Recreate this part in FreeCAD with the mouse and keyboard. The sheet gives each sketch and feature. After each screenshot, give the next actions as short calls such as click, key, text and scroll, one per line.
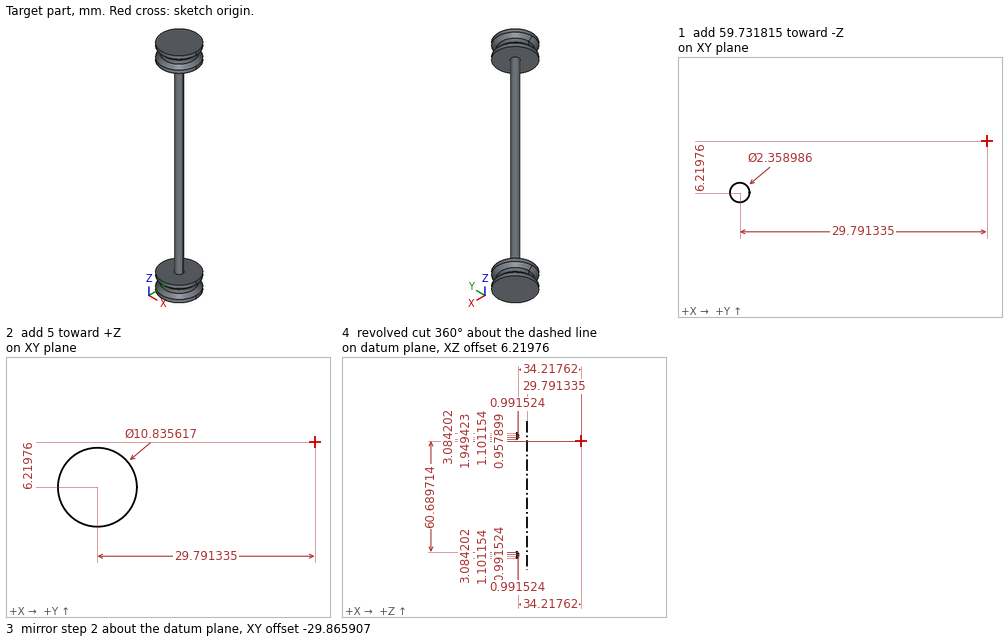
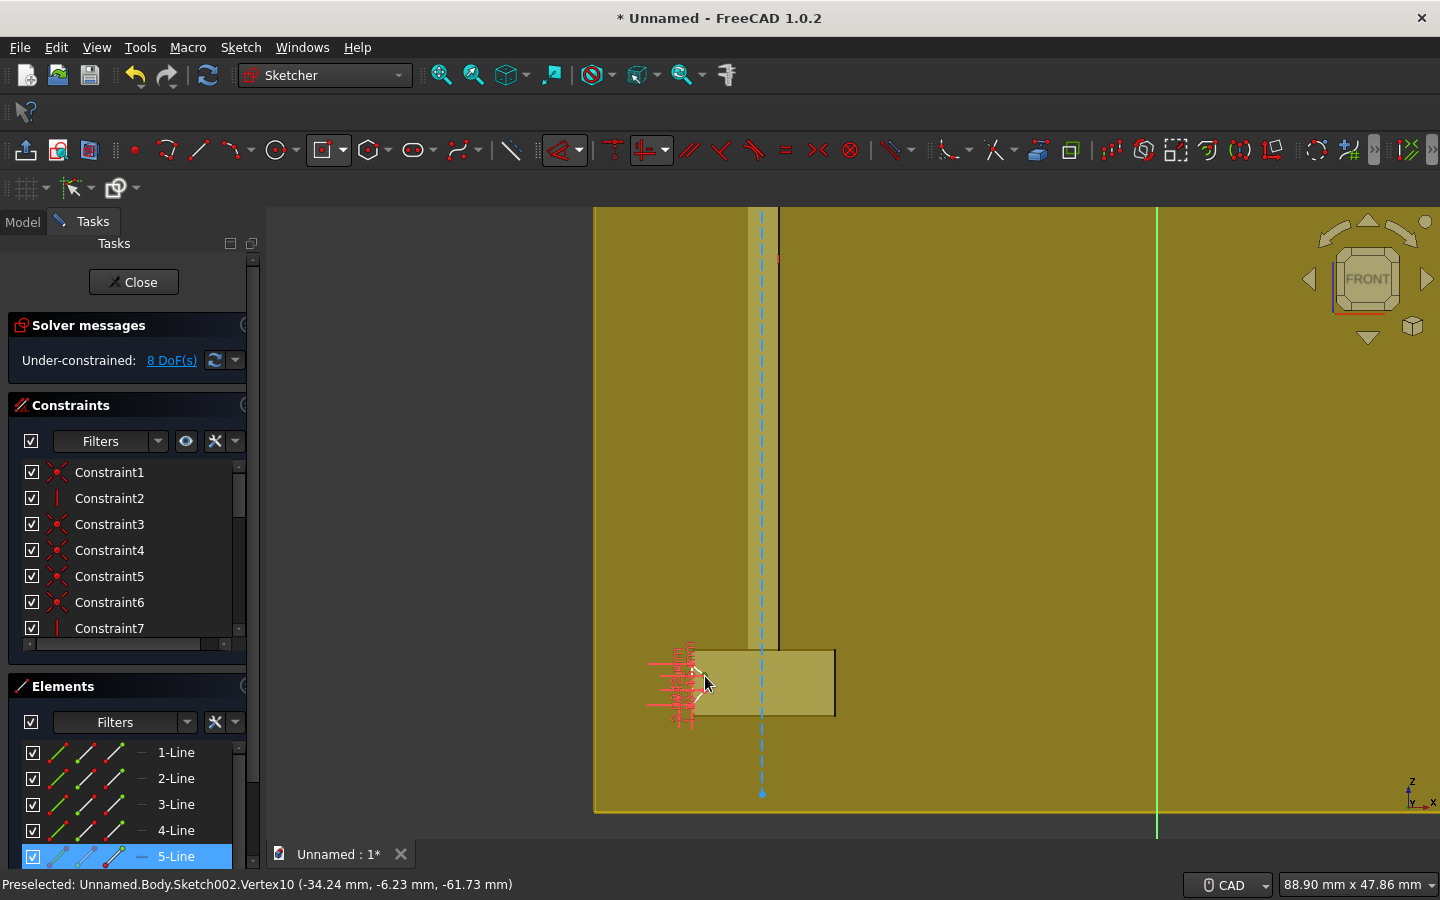
key(l)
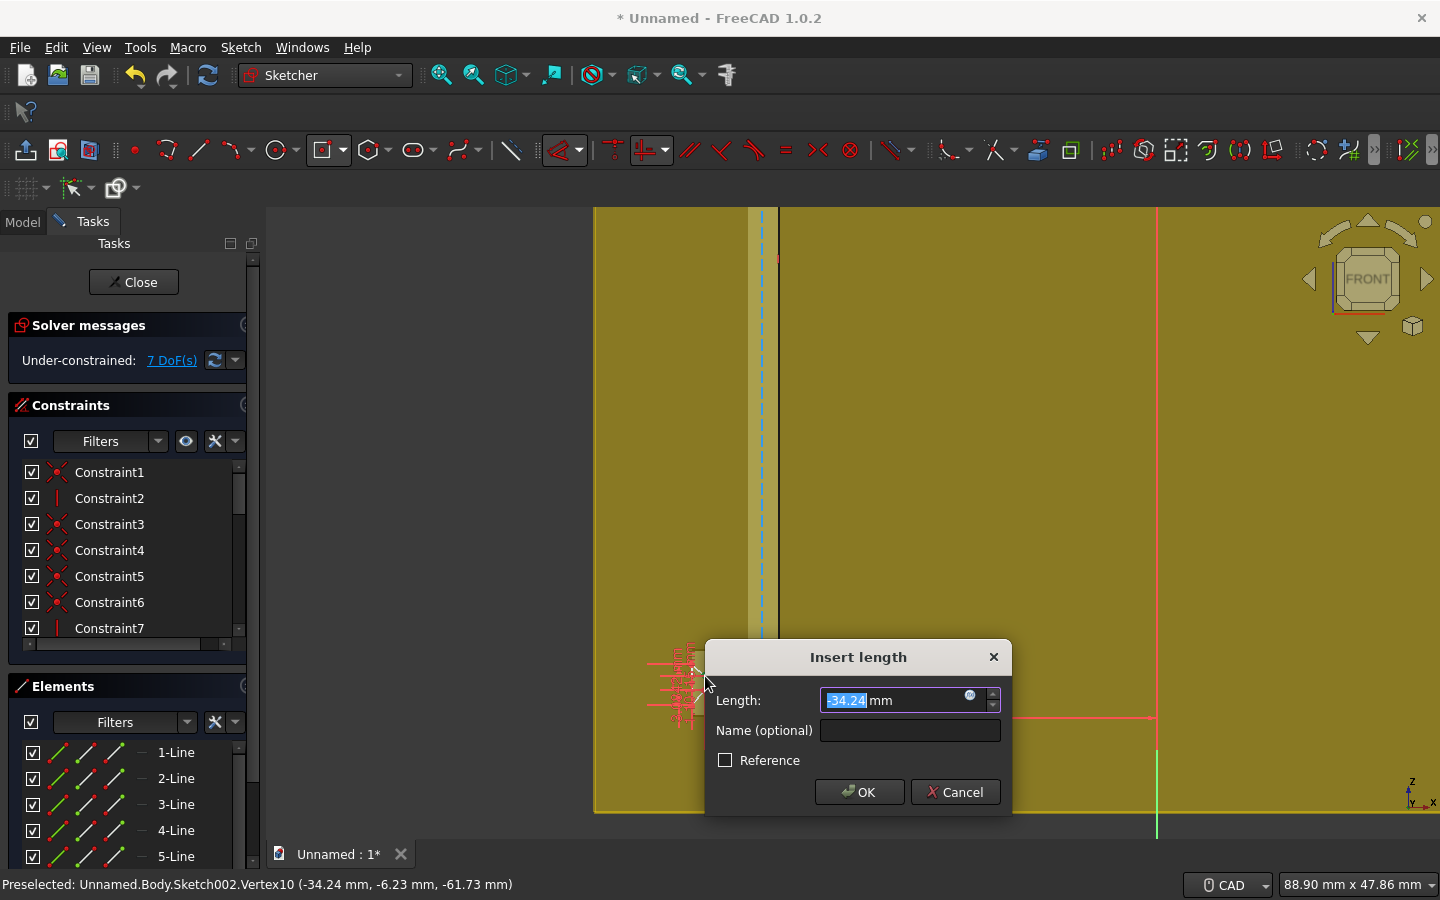
text(-34.21762)
key(Return)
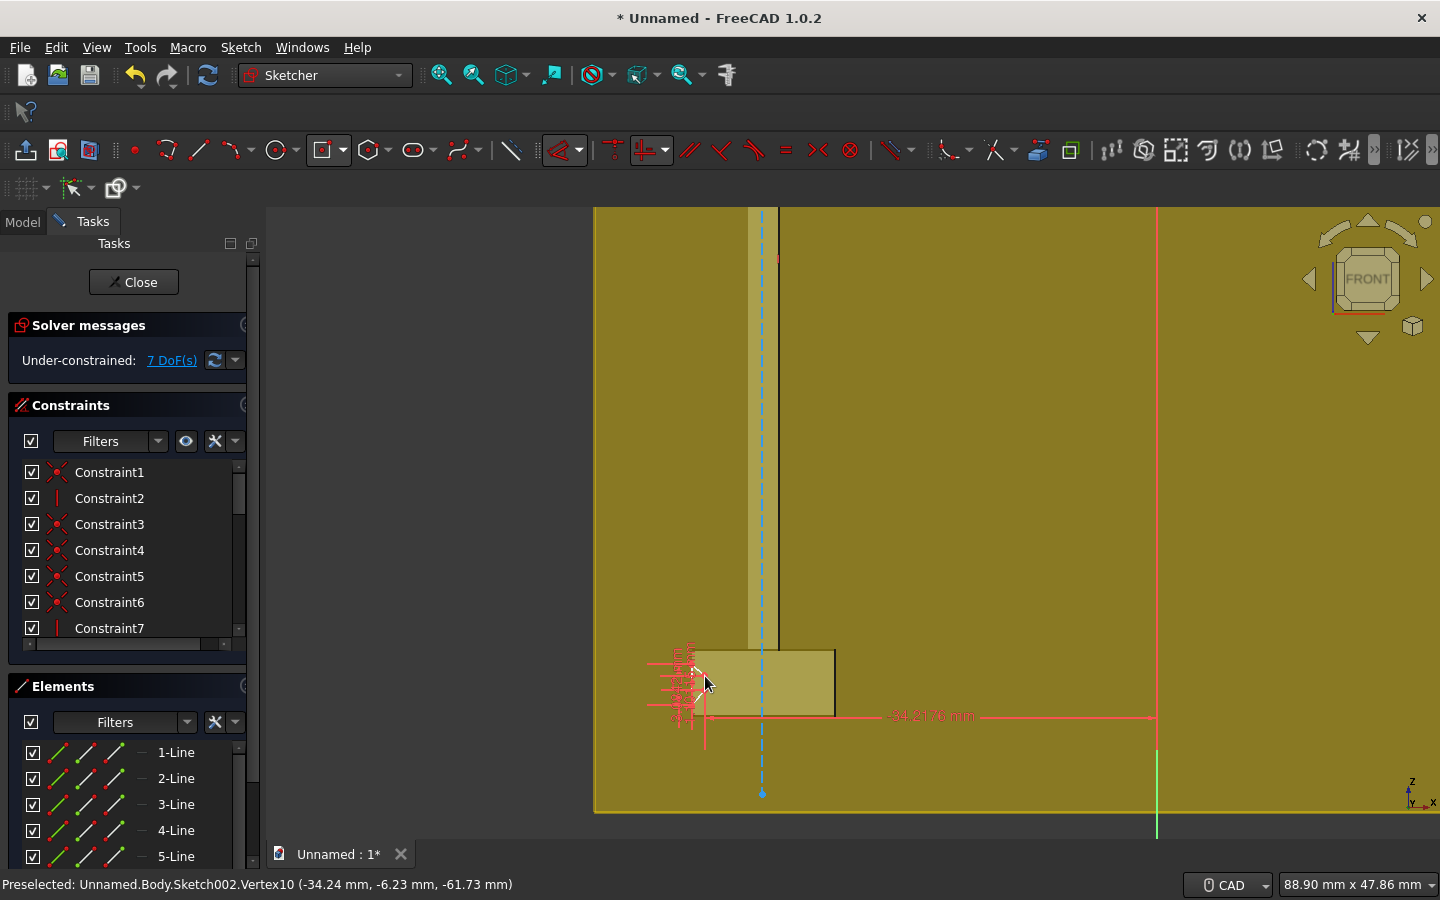
scroll(703, 679, down, 5)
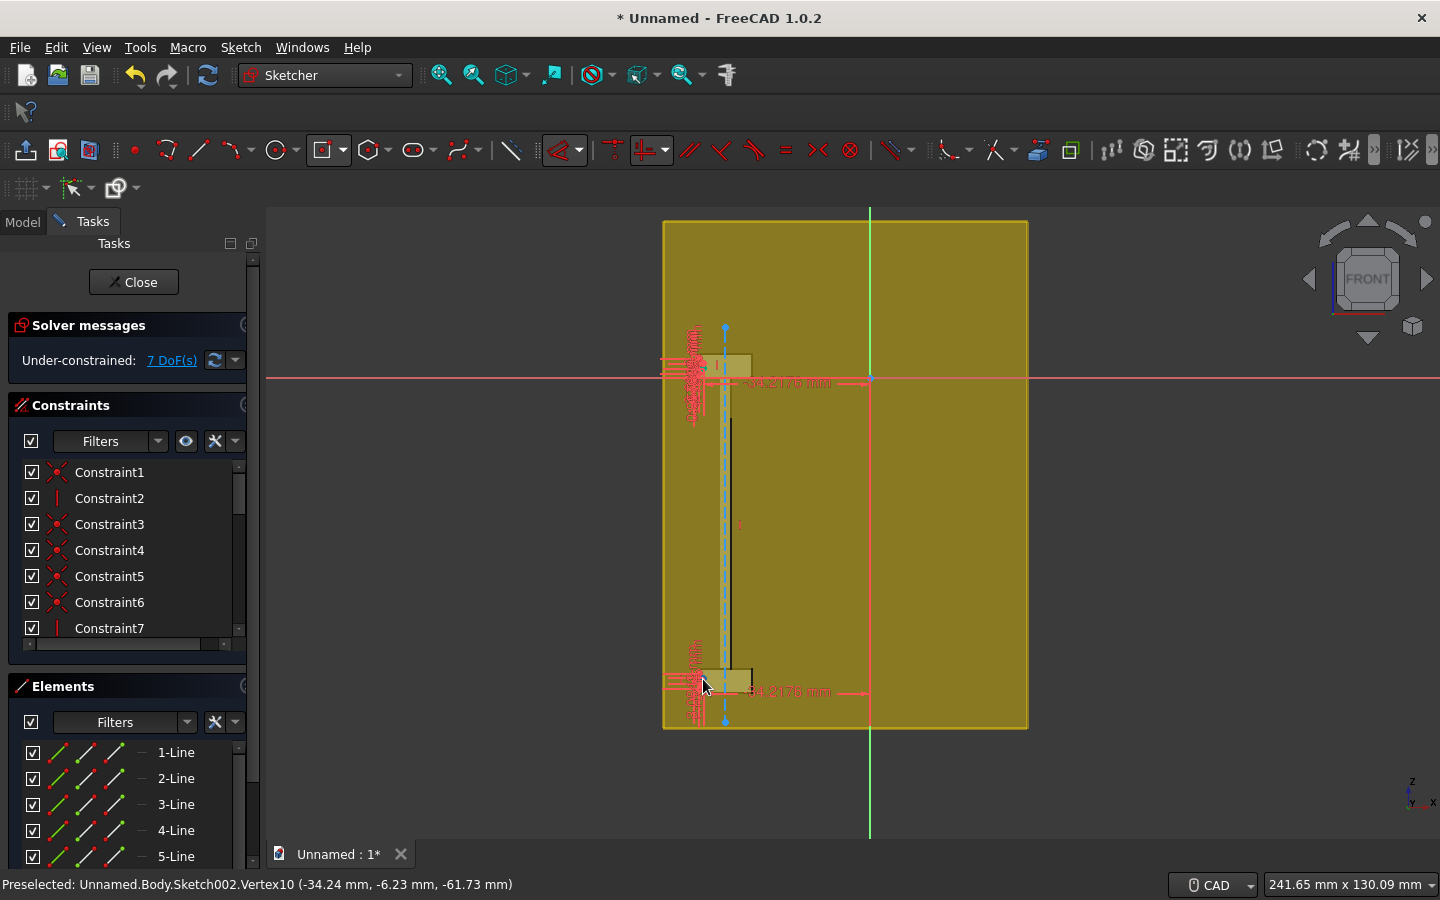
scroll(702, 371, up, 11)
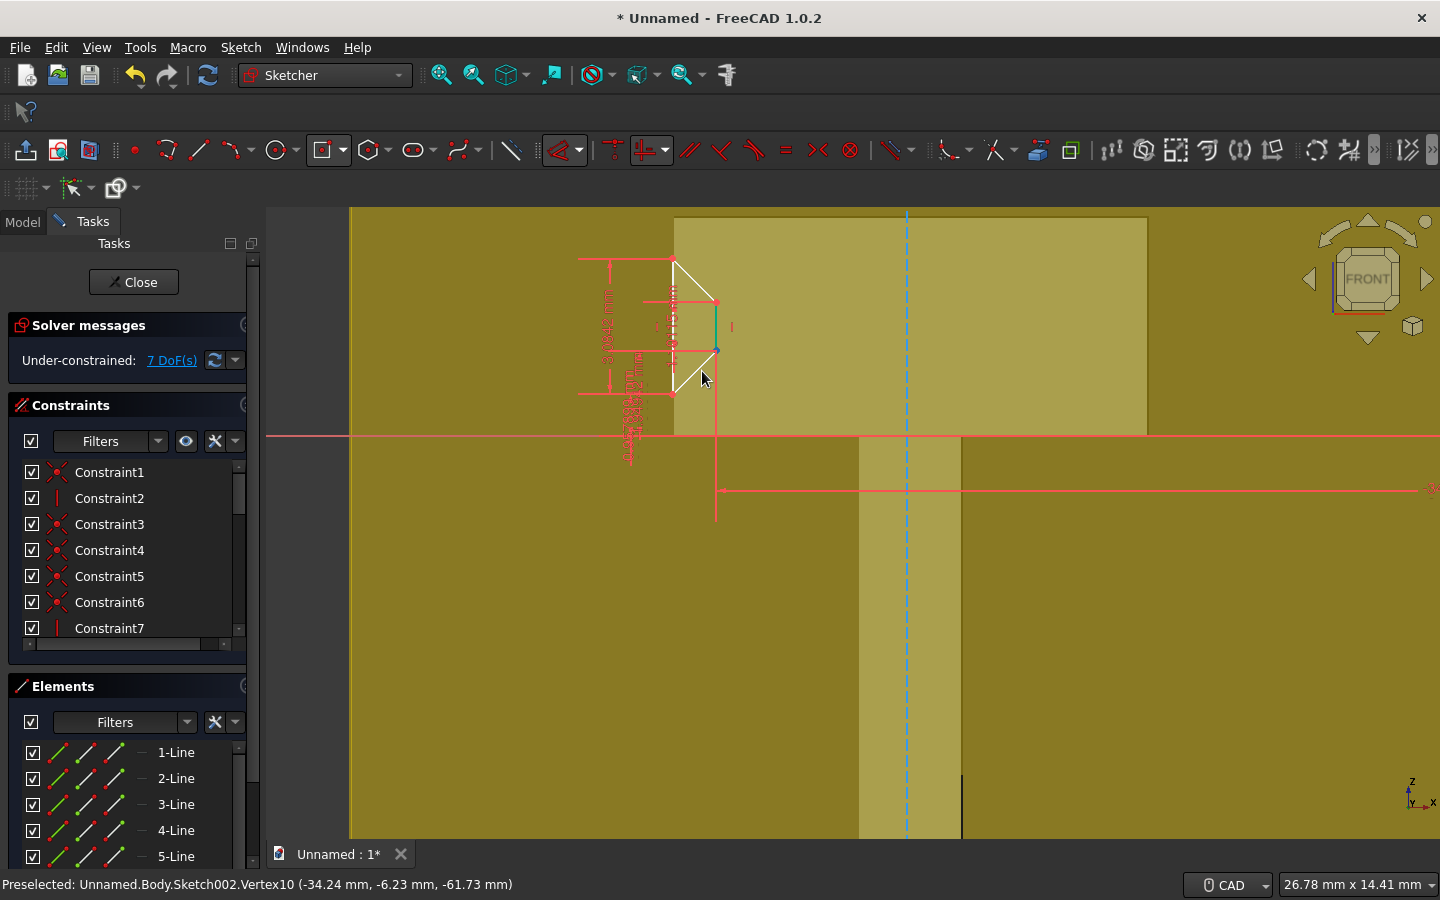
click(699, 368)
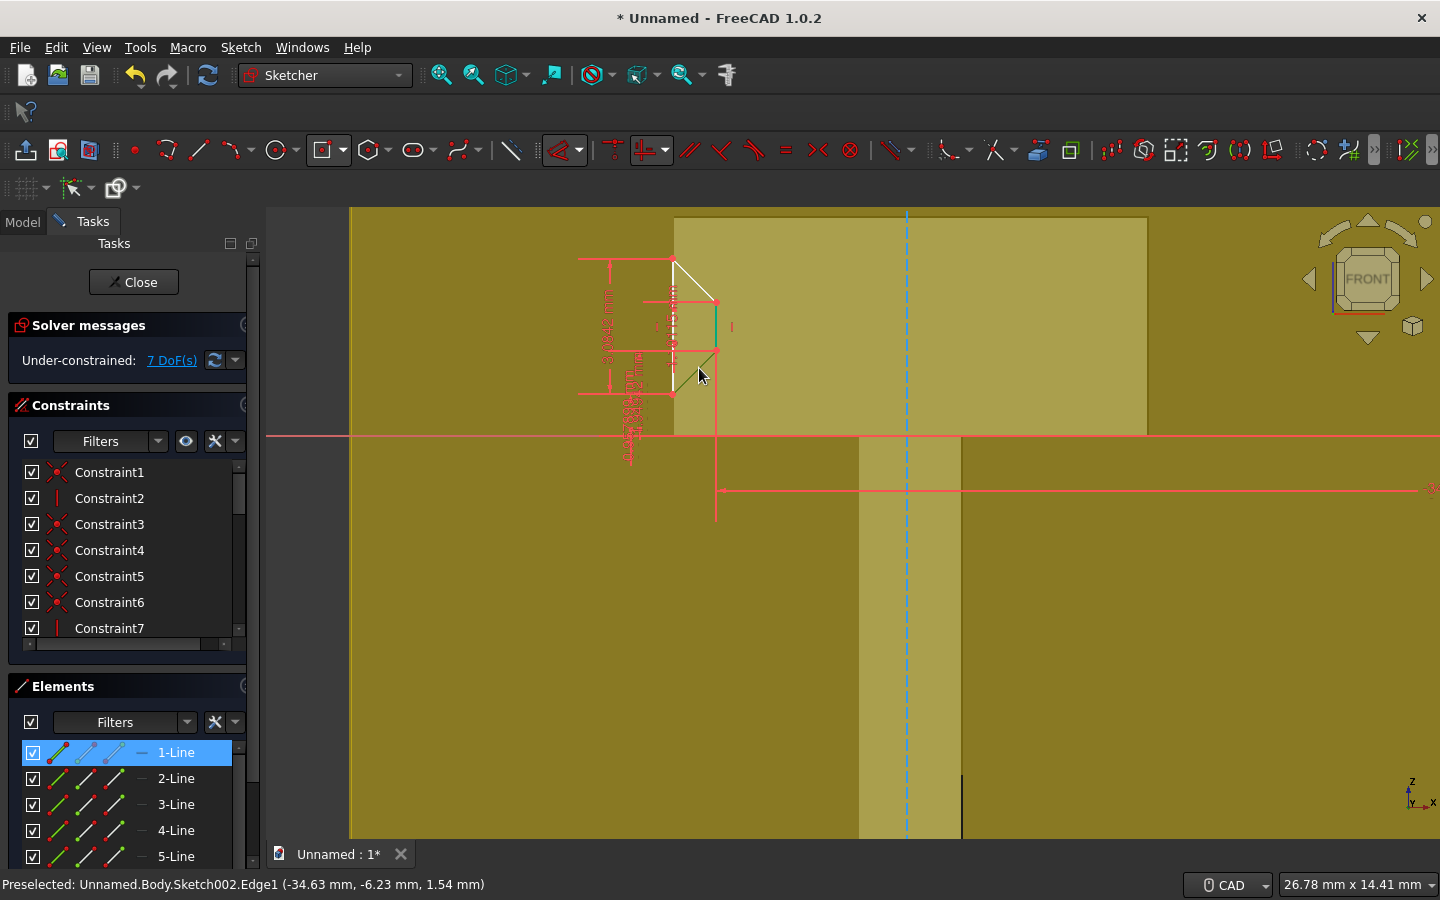
key(l)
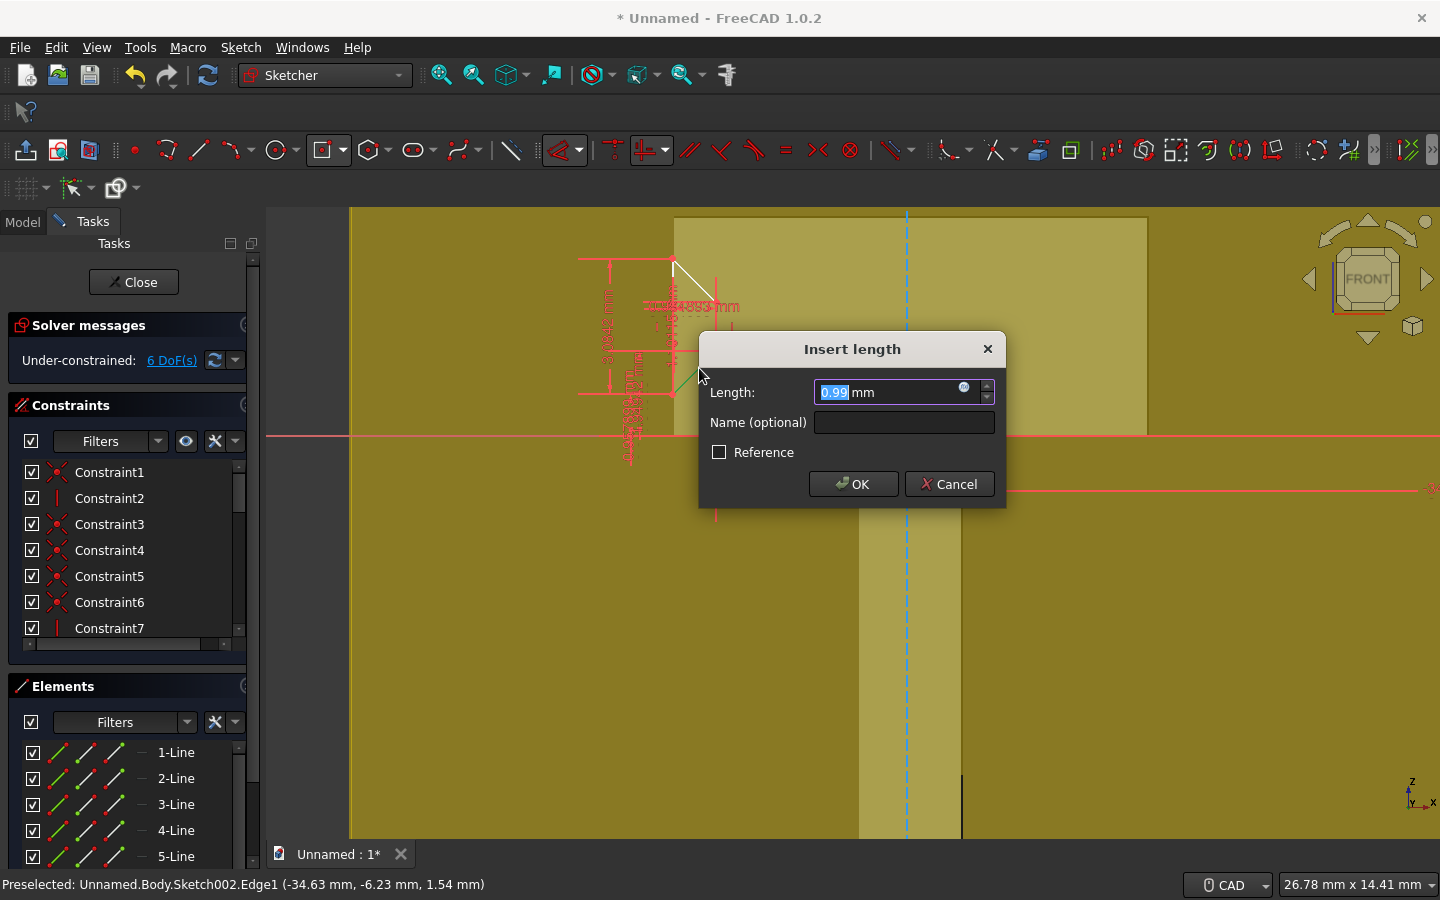
text(0.991524)
key(Return)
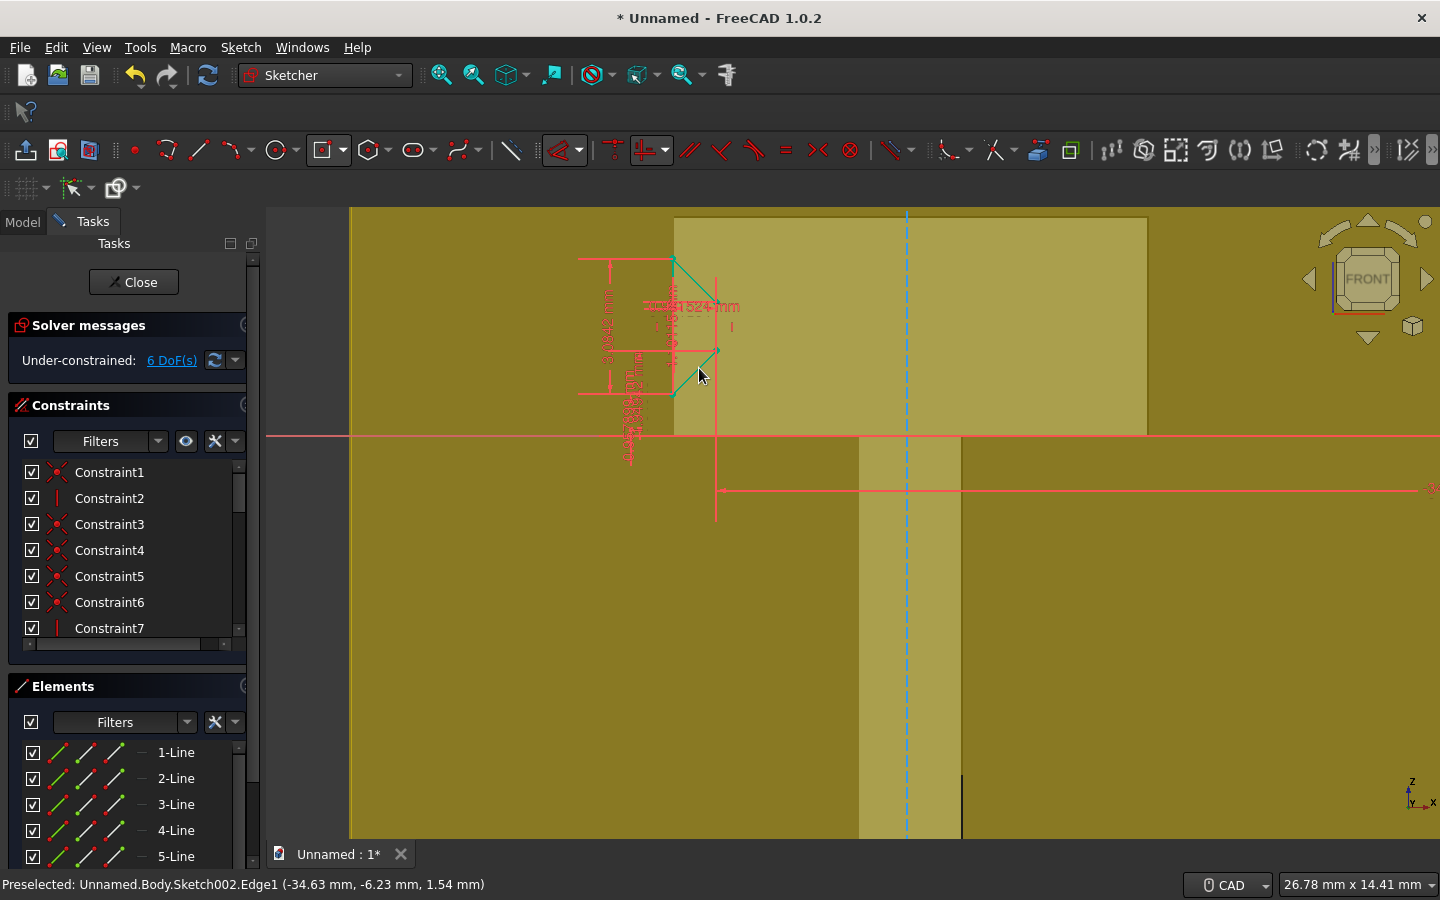
scroll(702, 371, down, 11)